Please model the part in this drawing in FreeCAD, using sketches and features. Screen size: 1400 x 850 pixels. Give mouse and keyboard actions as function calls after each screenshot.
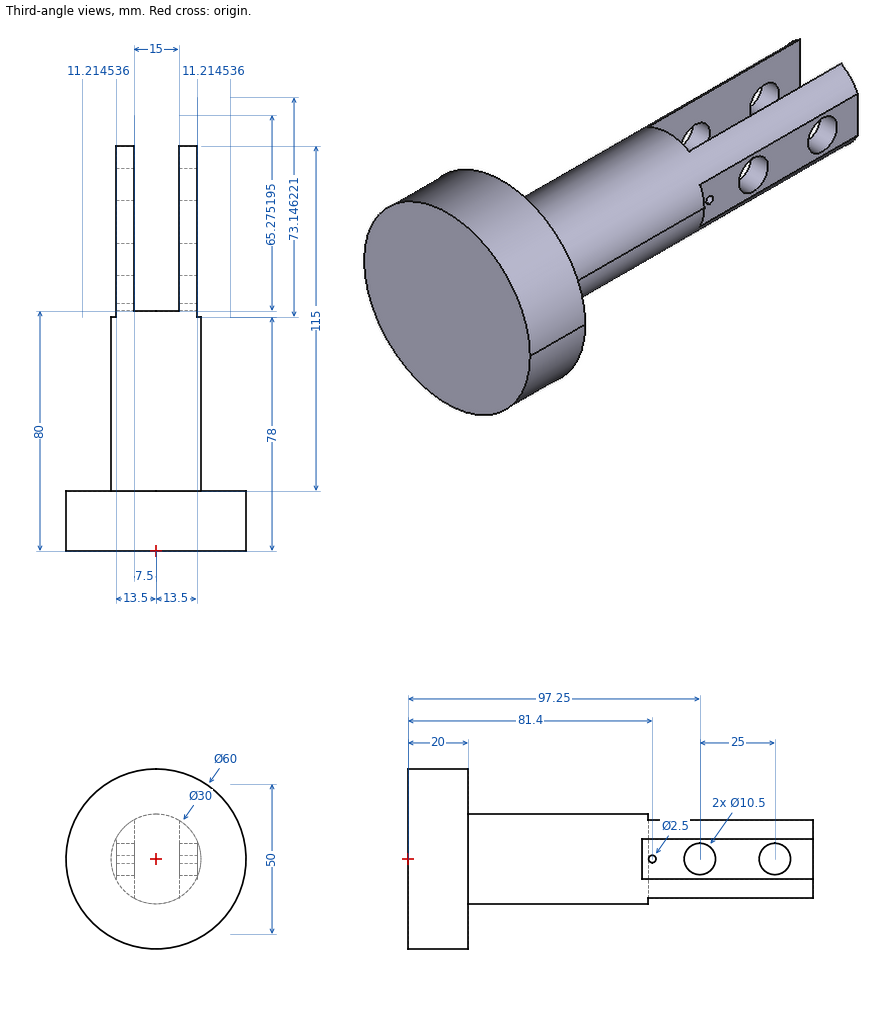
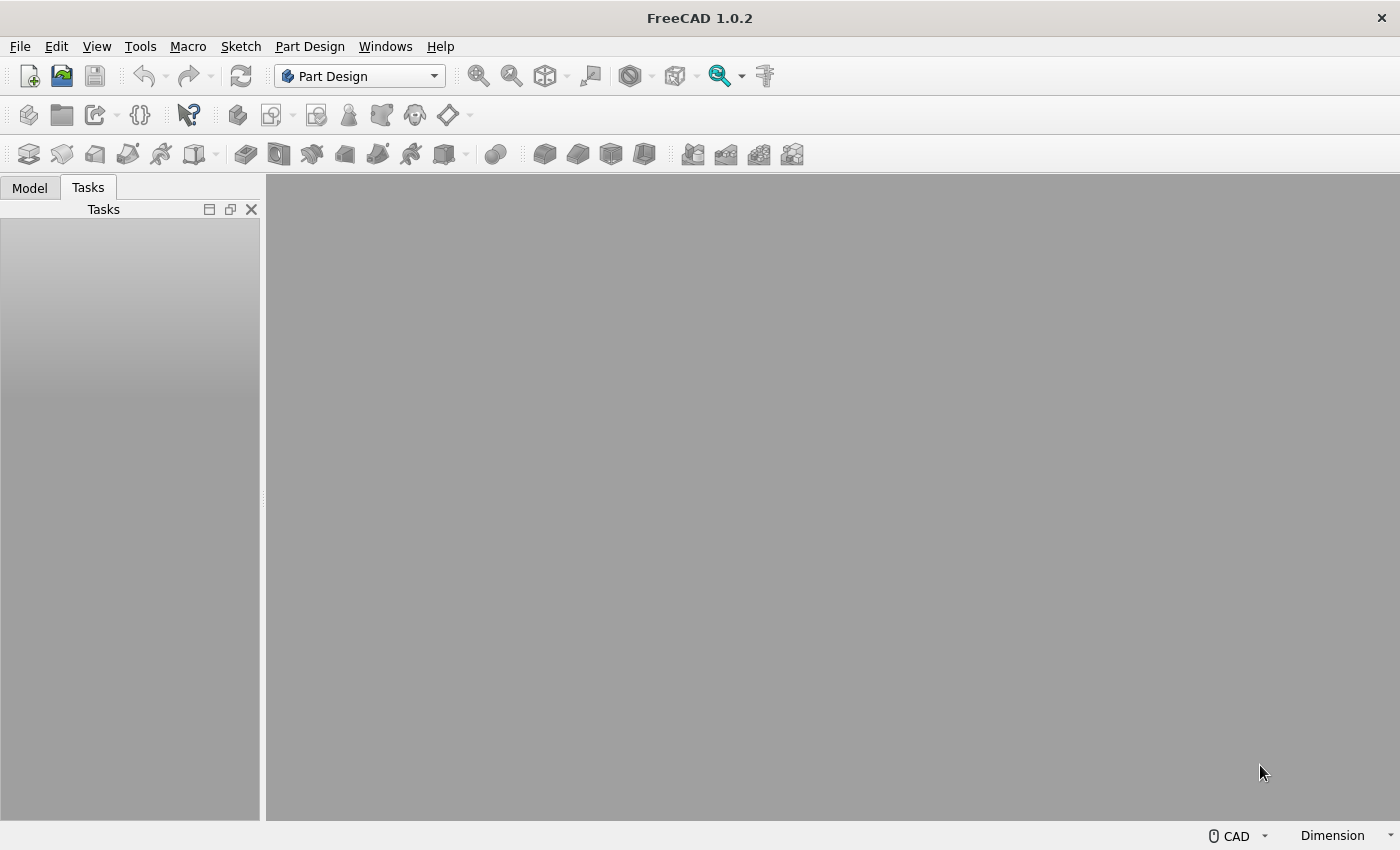
click(29, 76)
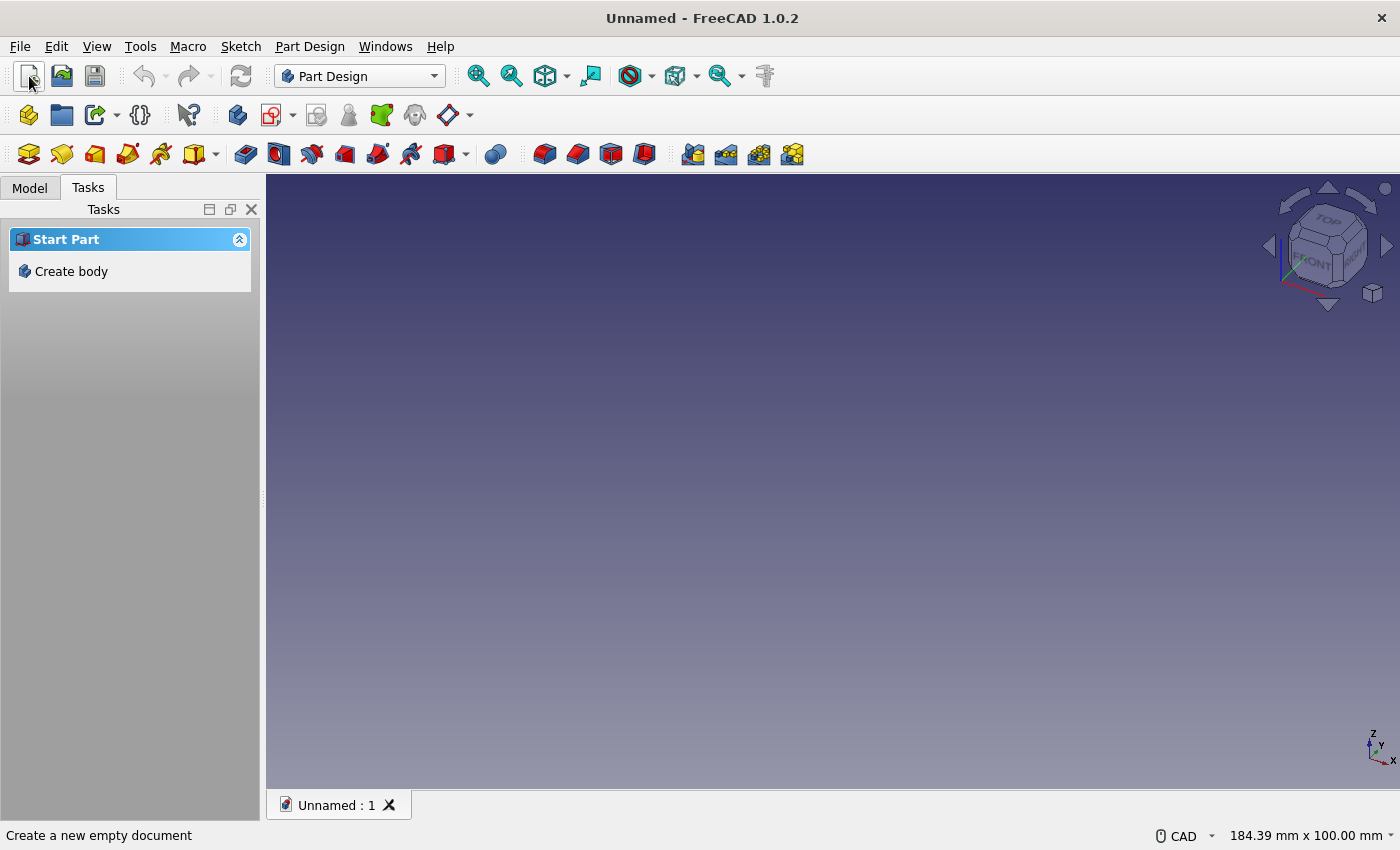
click(270, 116)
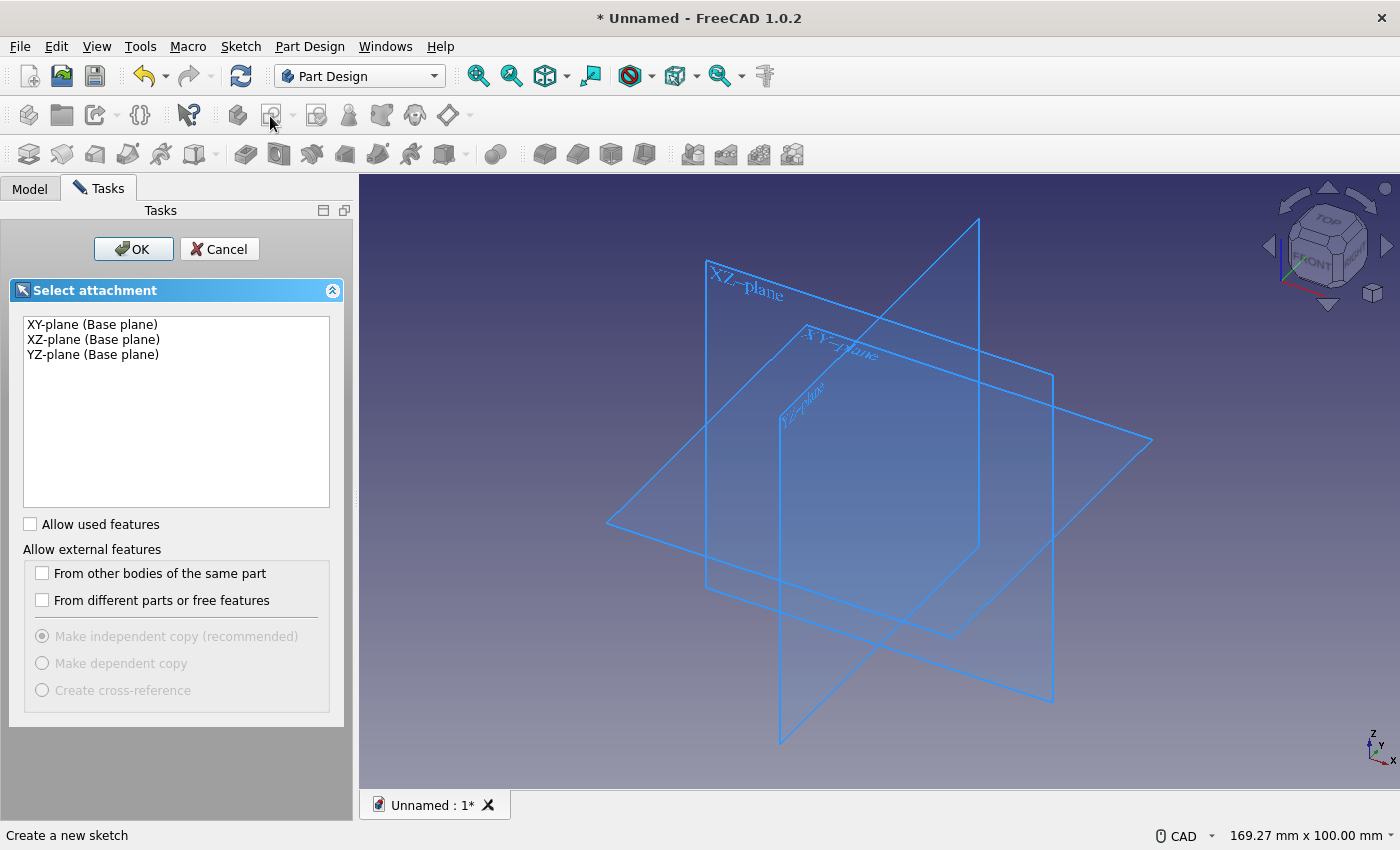
click(84, 340)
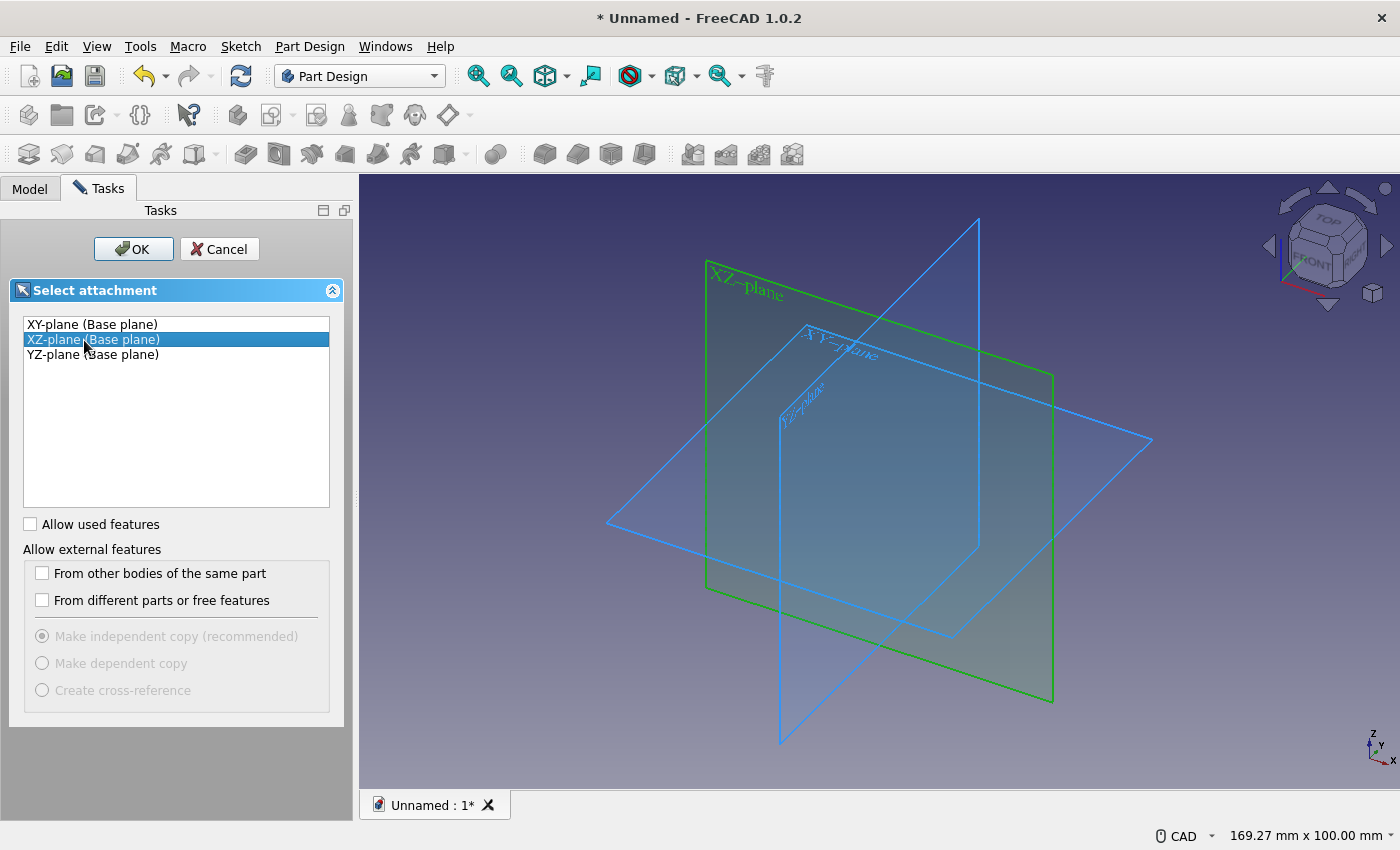
click(134, 249)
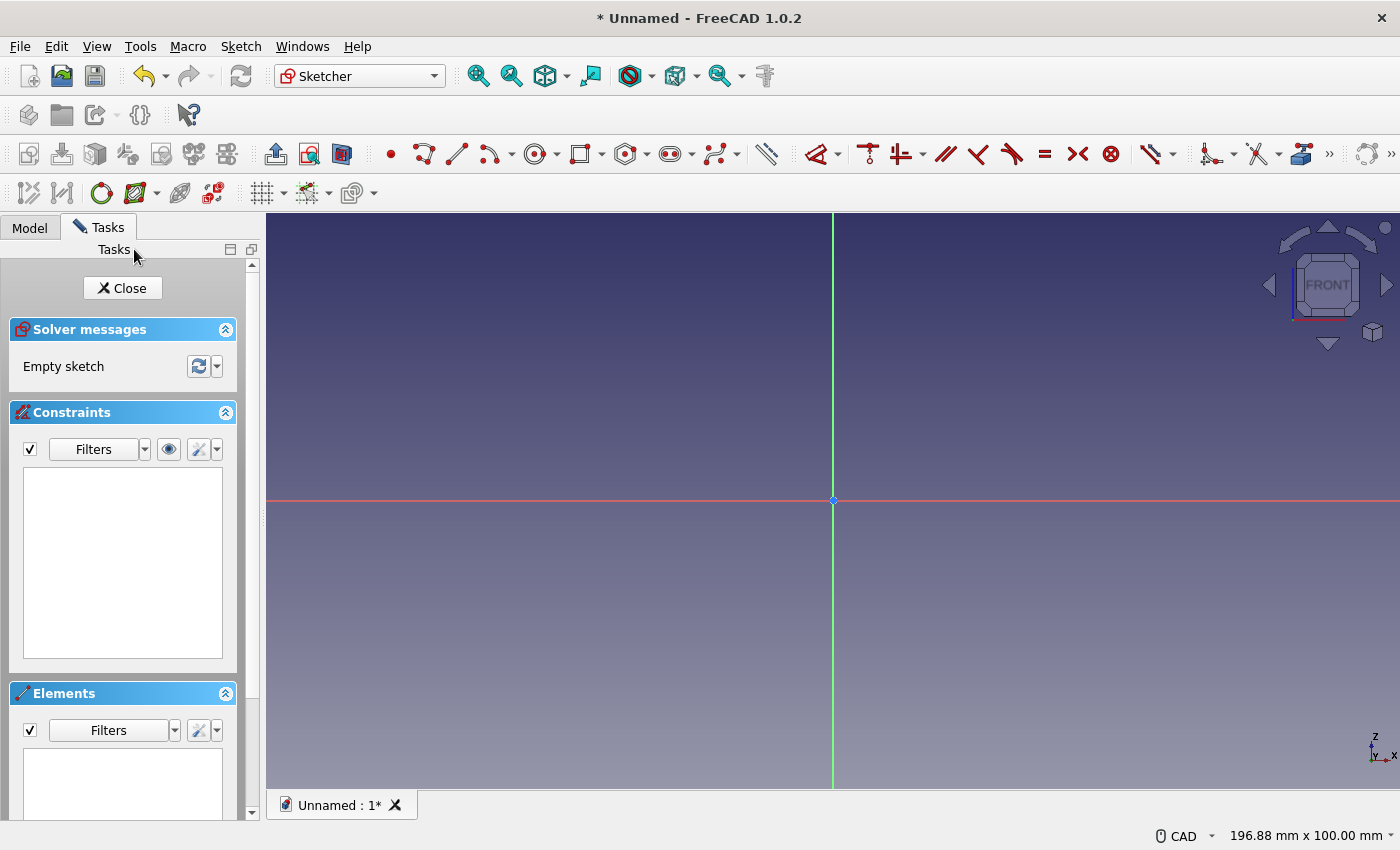
click(534, 154)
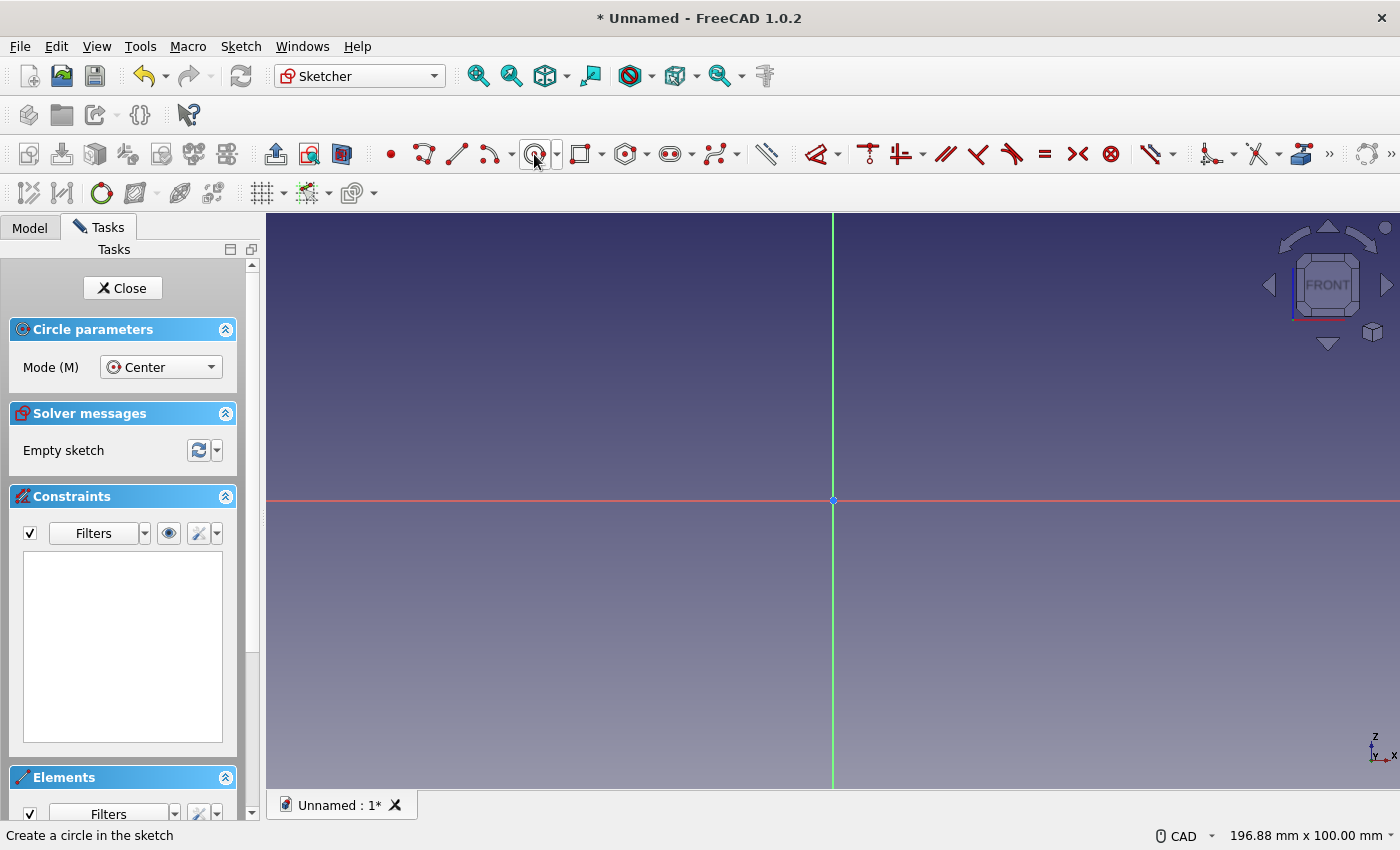
click(833, 501)
move(955, 379)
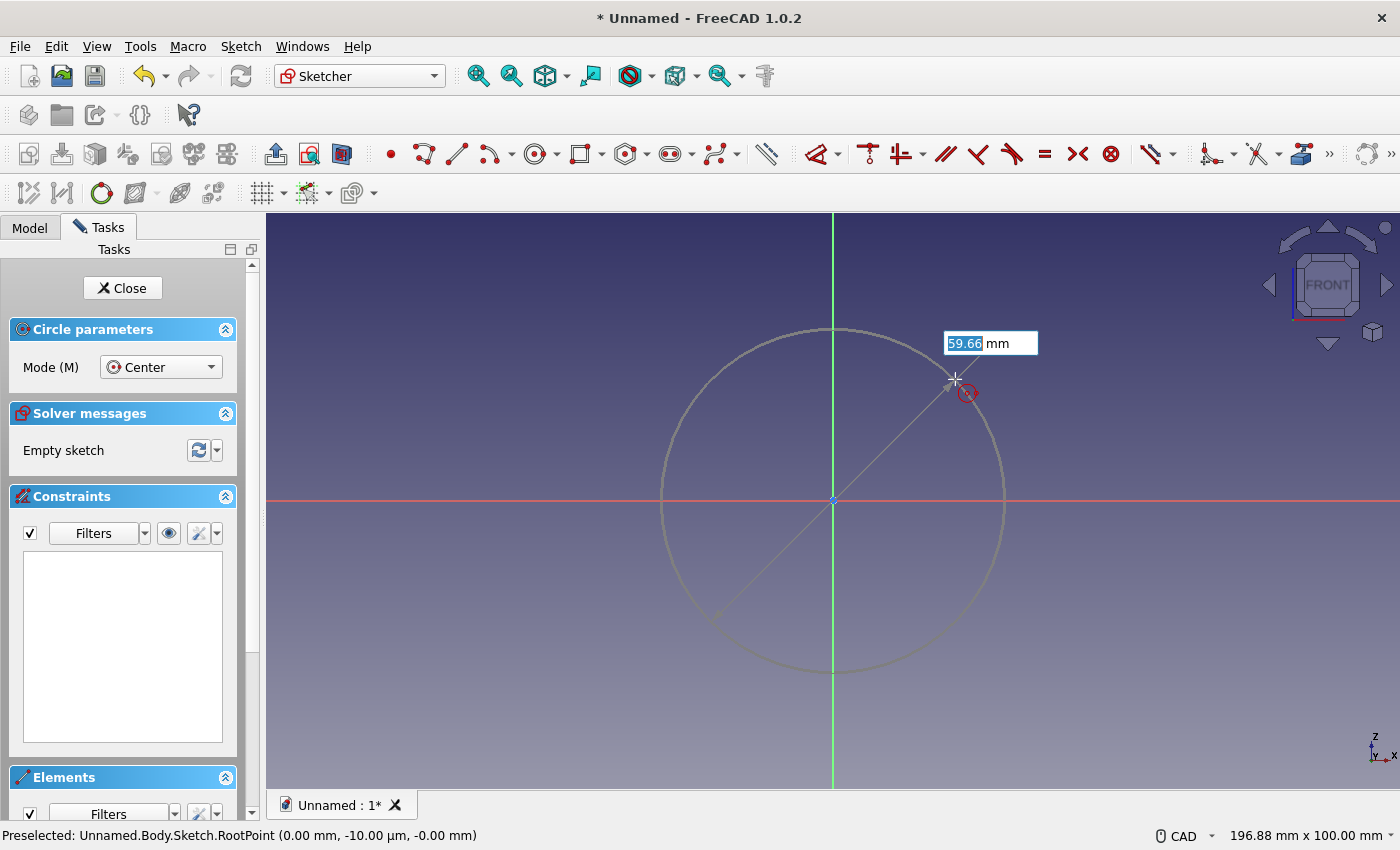
text(60)
key(Return)
key(Escape)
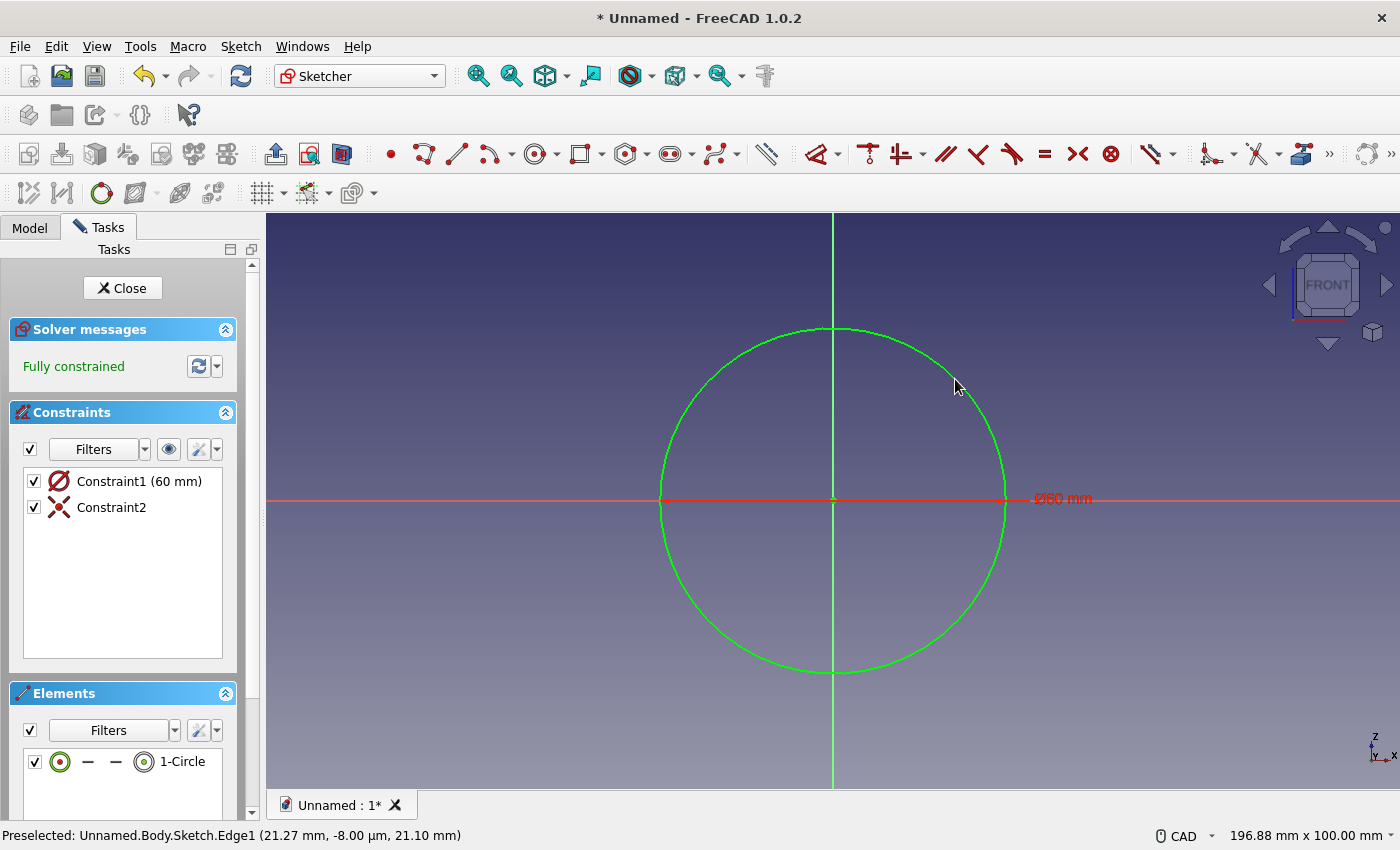
click(123, 288)